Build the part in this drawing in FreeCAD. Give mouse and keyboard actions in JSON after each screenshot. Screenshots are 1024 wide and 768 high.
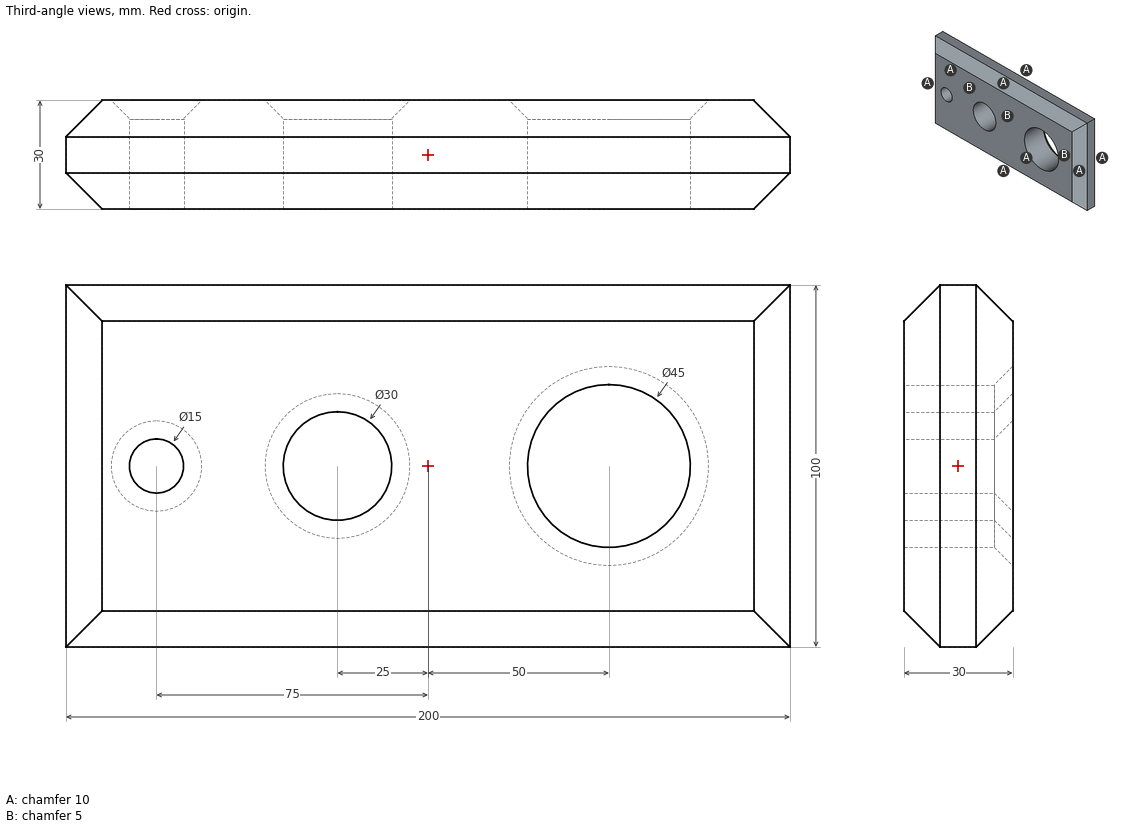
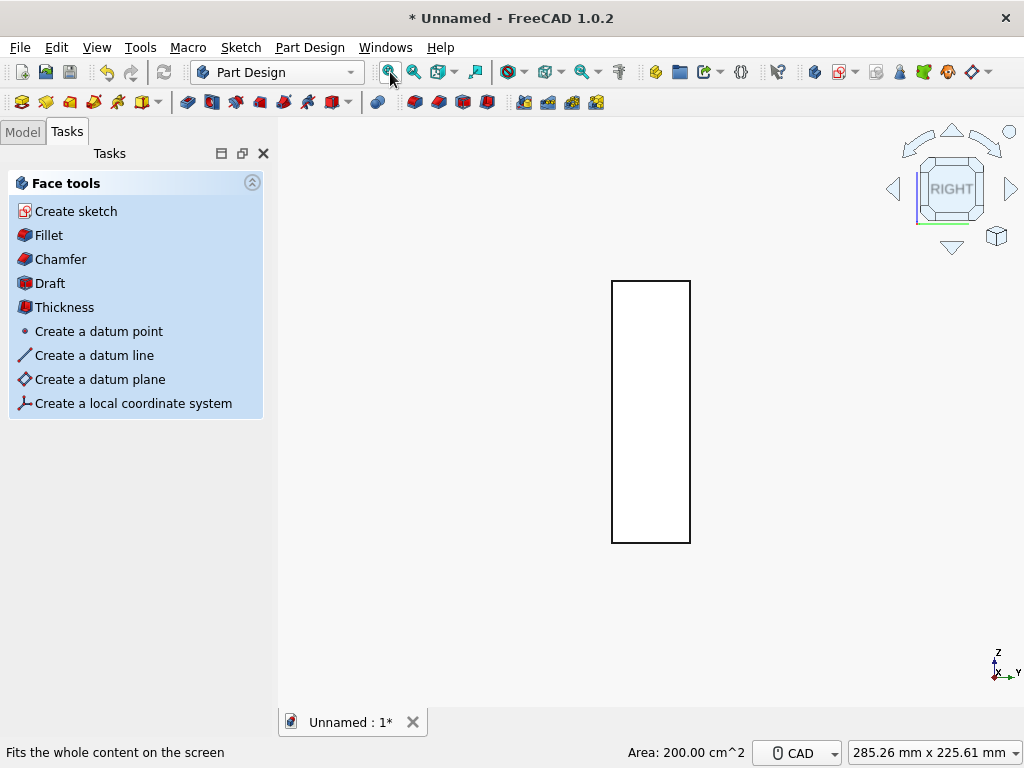
{"action": "key", "text": "5"}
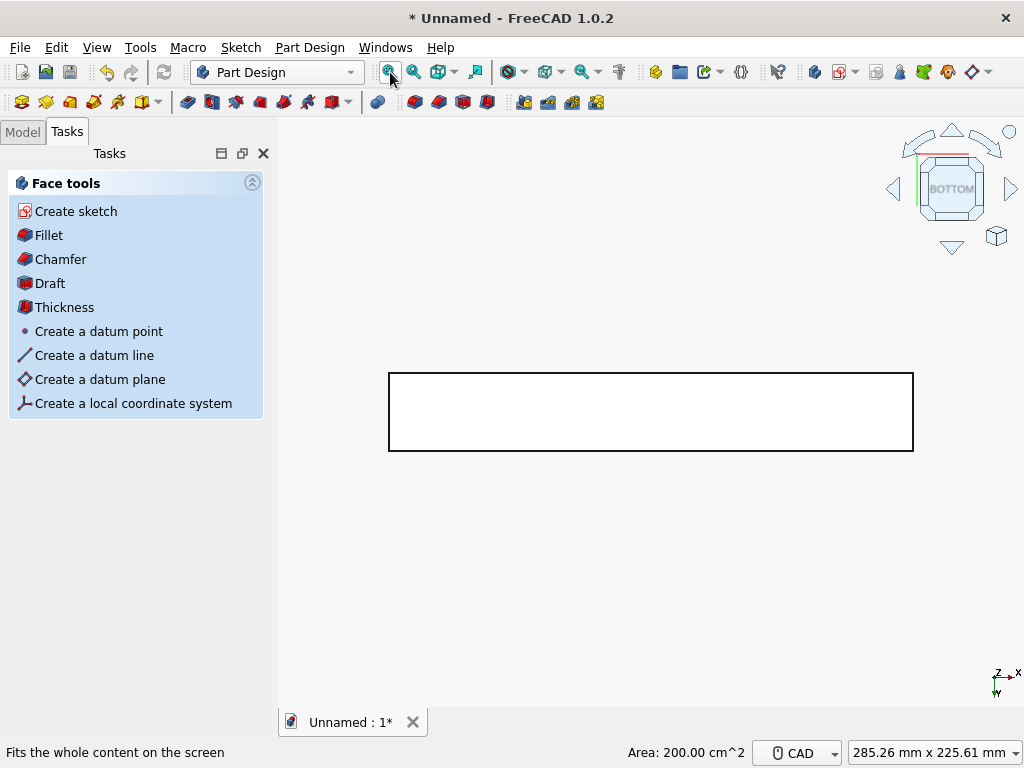
{"action": "key", "text": "4"}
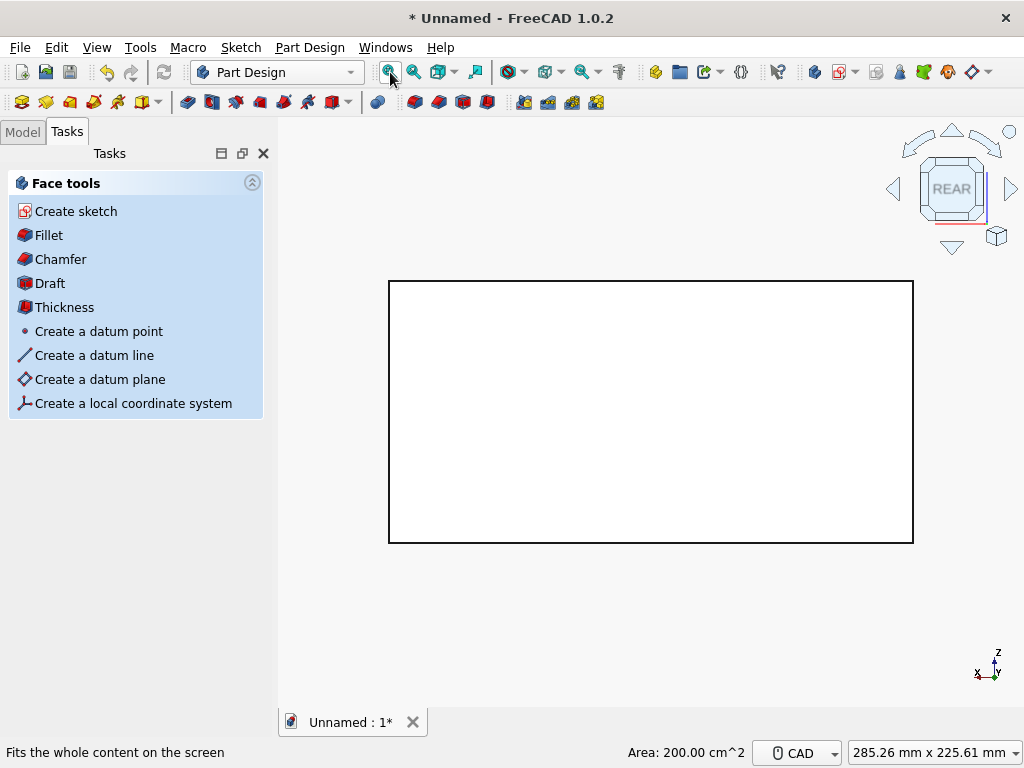
{"action": "left_click", "coordinate": [576, 411], "text": "ctrl"}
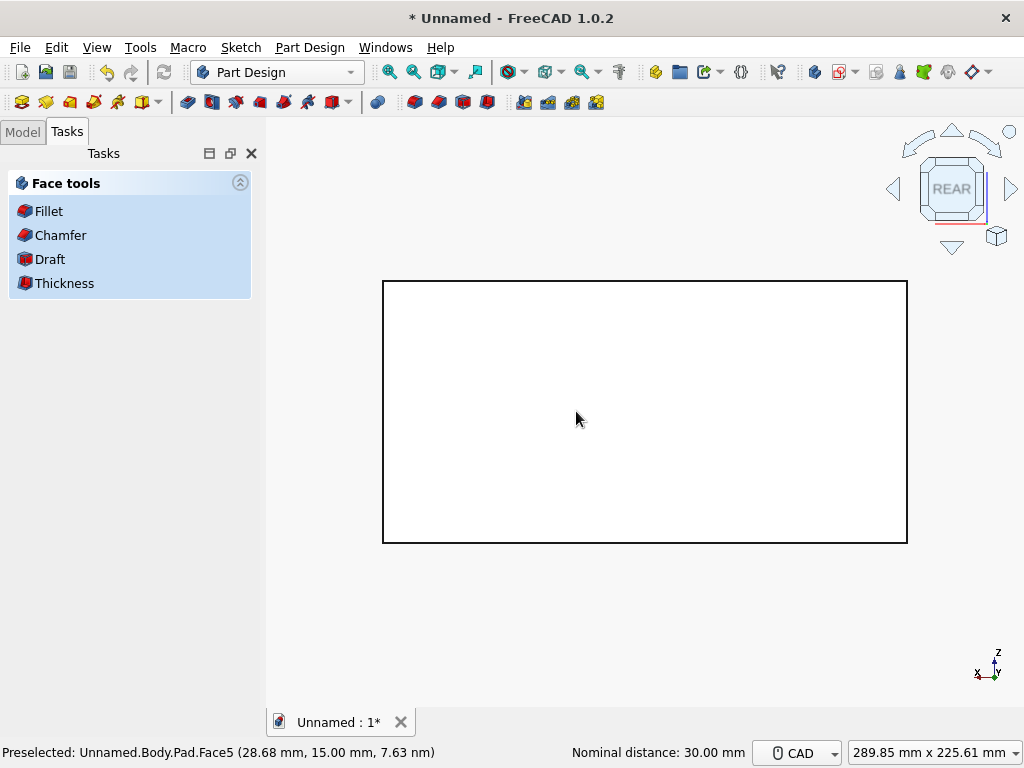
{"action": "left_click", "coordinate": [440, 102]}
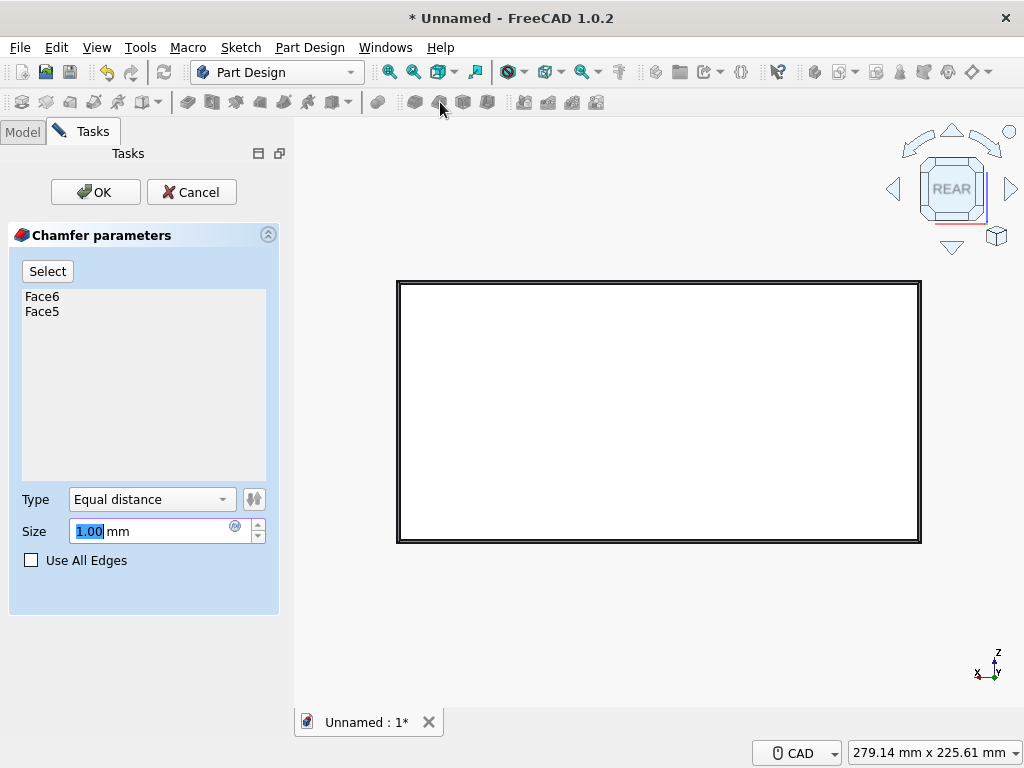
{"action": "type", "text": "10"}
{"action": "key", "text": "Tab"}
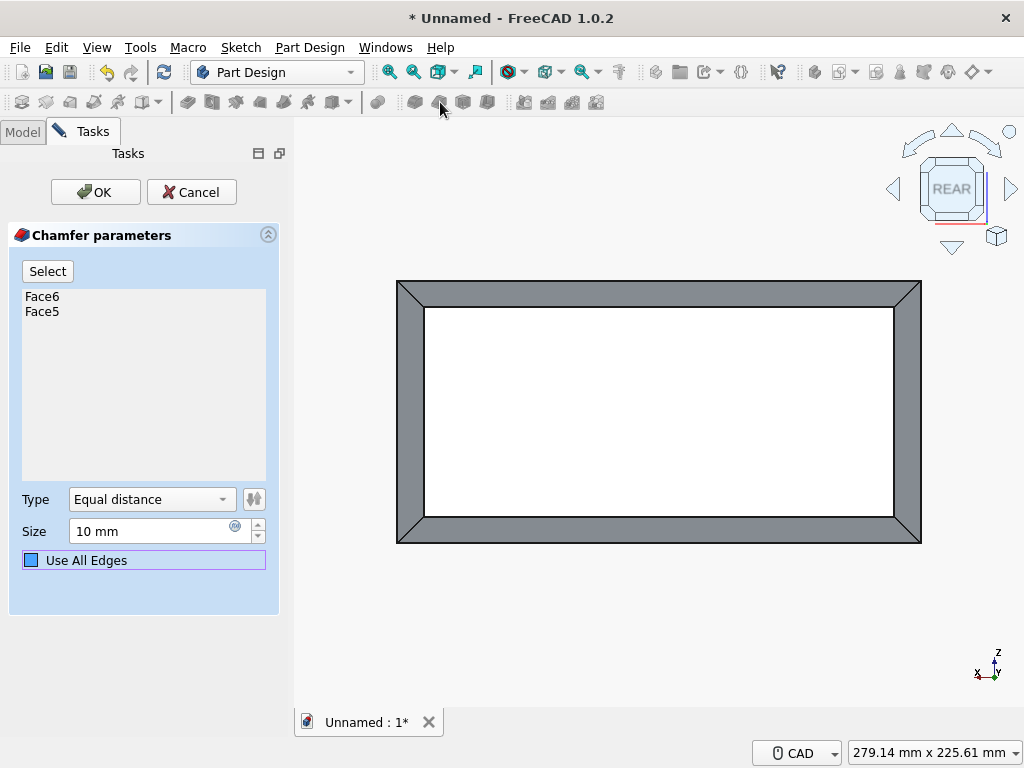
{"action": "left_click", "coordinate": [96, 192]}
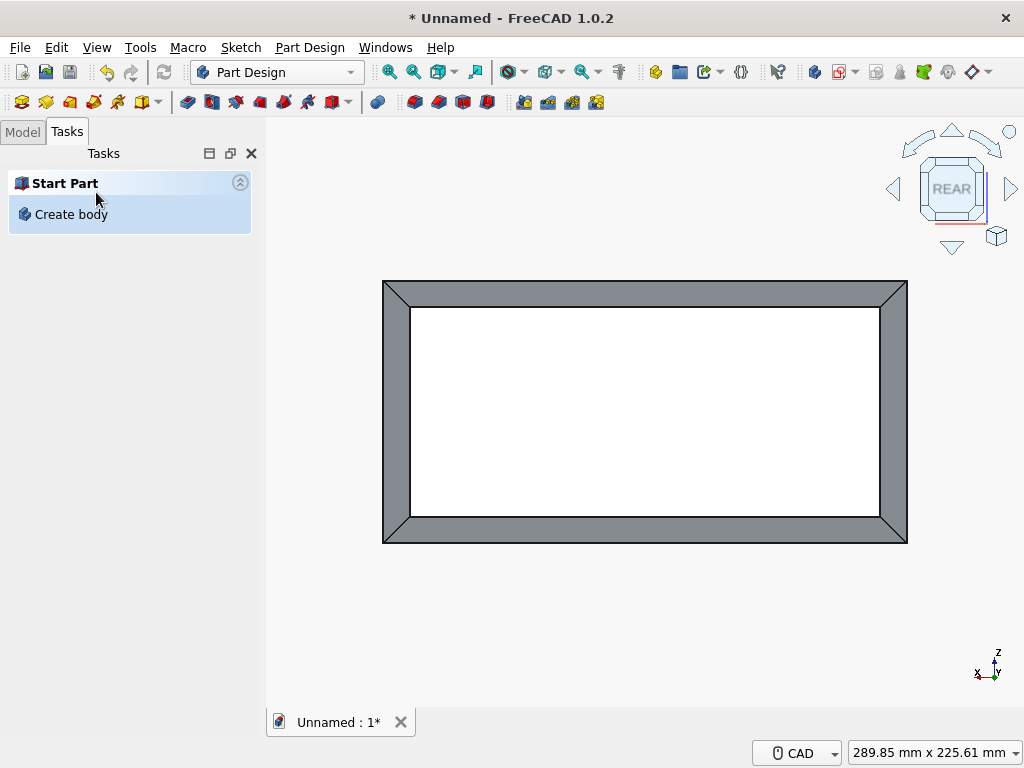
{"action": "left_click", "coordinate": [578, 411]}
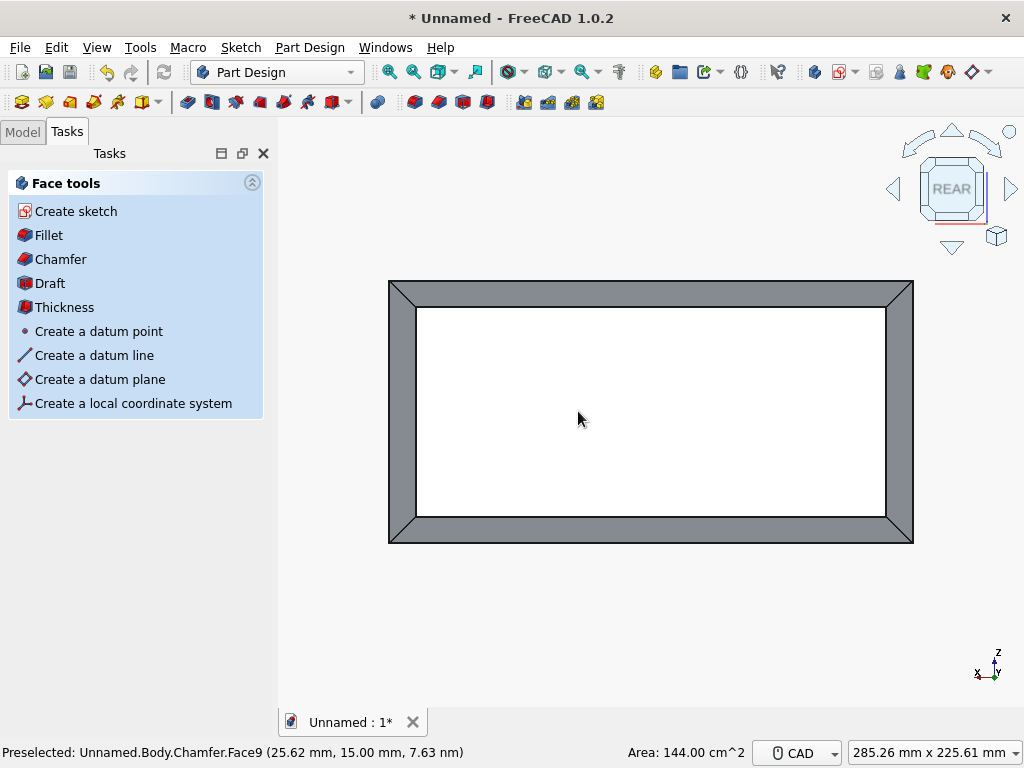
{"action": "left_click", "coordinate": [840, 72]}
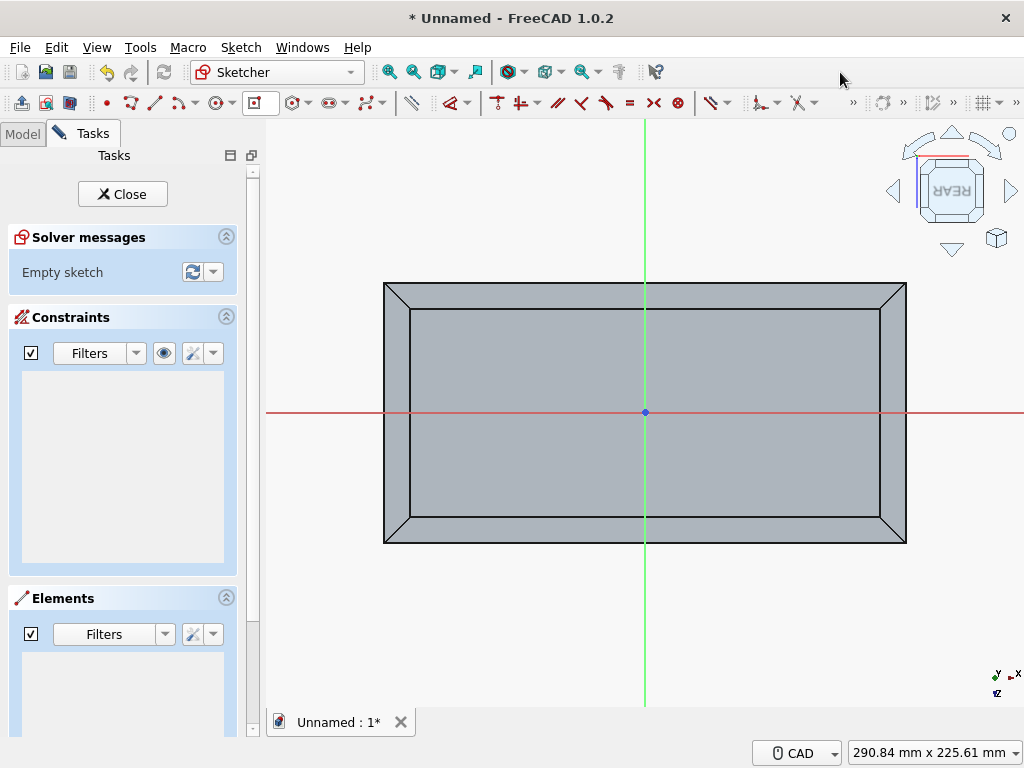
{"action": "left_click", "coordinate": [216, 104]}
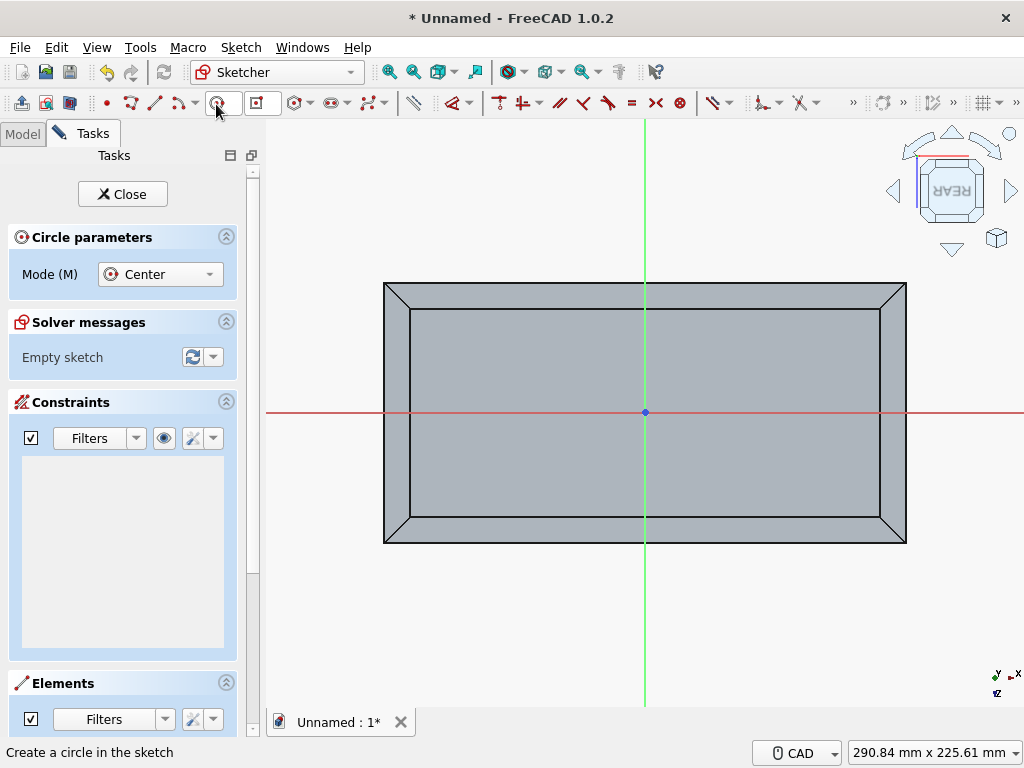
{"action": "left_click", "coordinate": [450, 413]}
{"action": "left_click", "coordinate": [456, 395]}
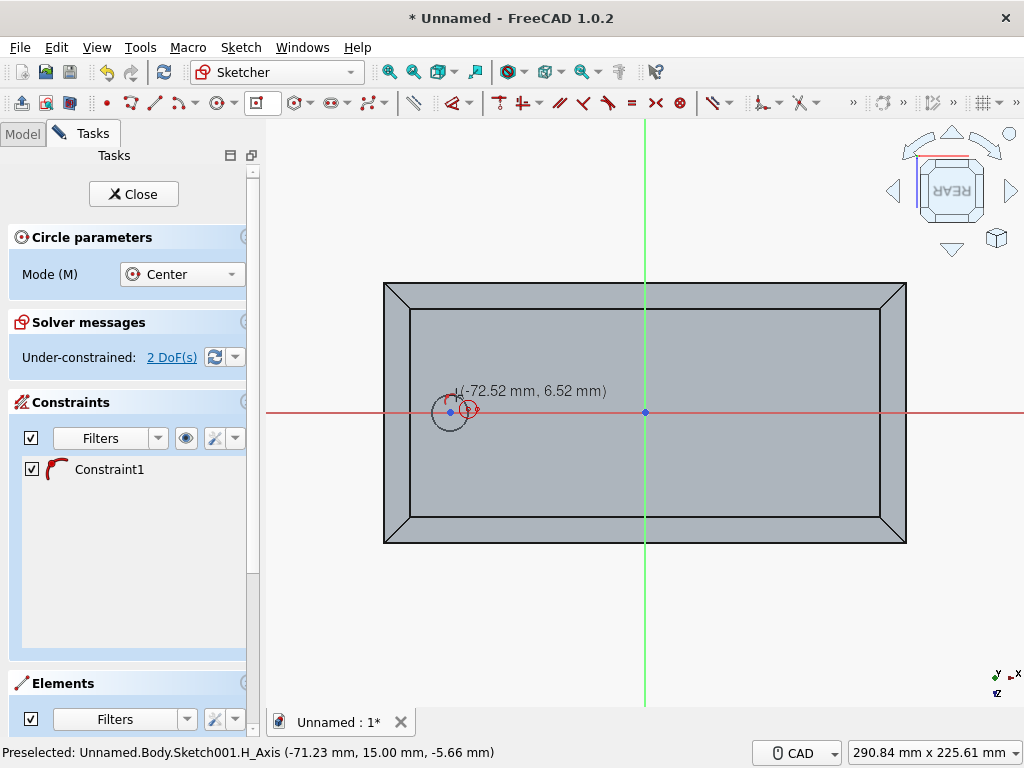
{"action": "left_click", "coordinate": [580, 413]}
{"action": "left_click", "coordinate": [607, 385]}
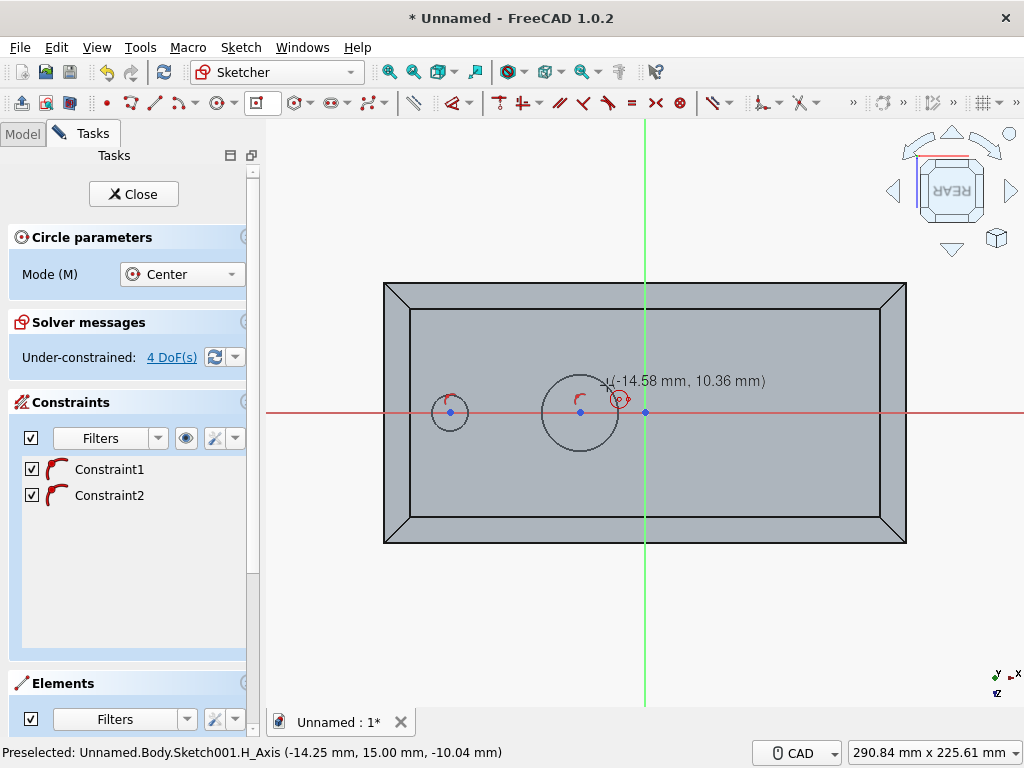
{"action": "left_click", "coordinate": [775, 413]}
{"action": "left_click", "coordinate": [817, 372]}
{"action": "key", "text": "Escape"}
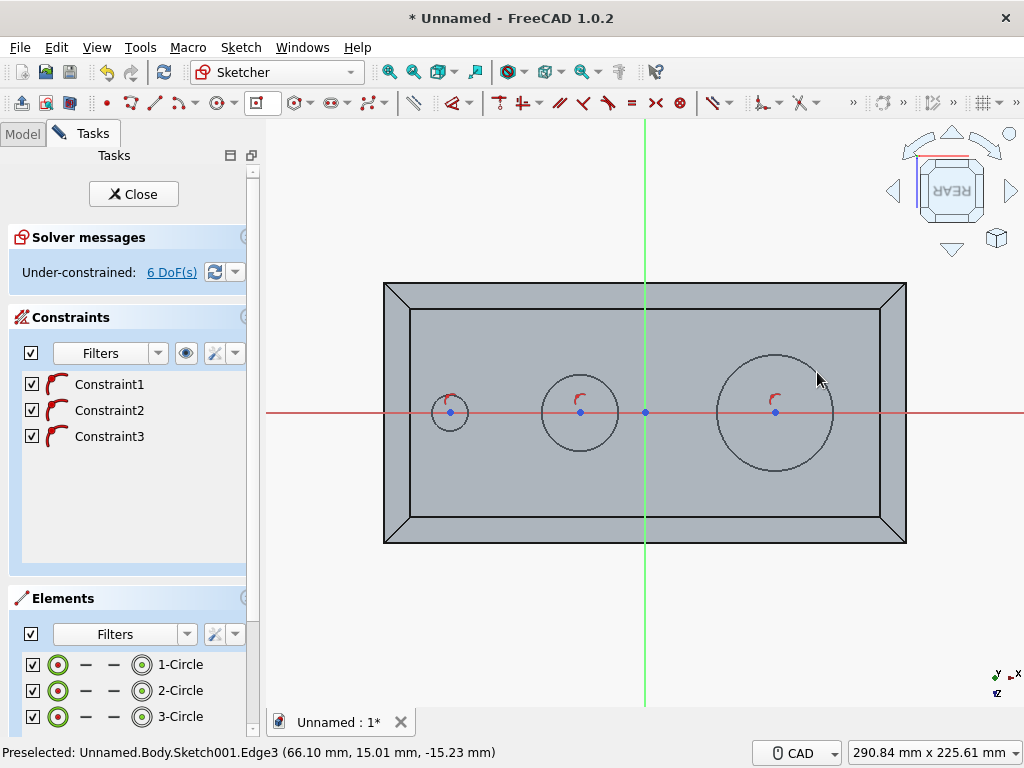
{"action": "left_click", "coordinate": [452, 104]}